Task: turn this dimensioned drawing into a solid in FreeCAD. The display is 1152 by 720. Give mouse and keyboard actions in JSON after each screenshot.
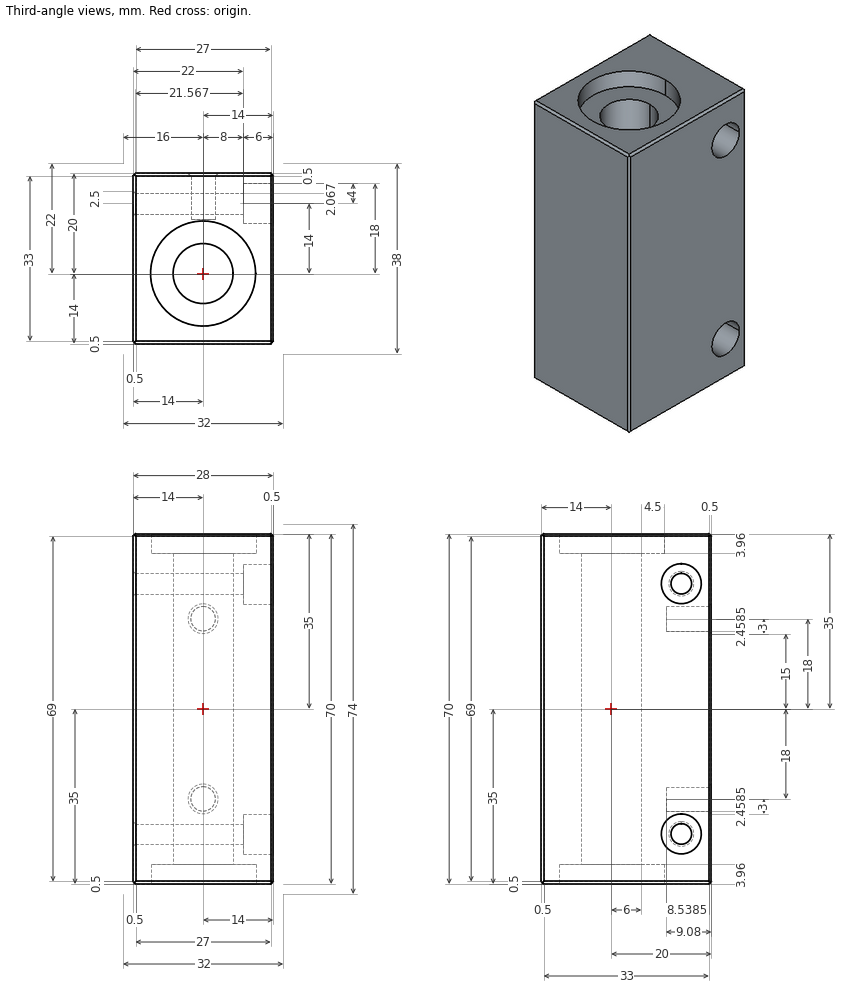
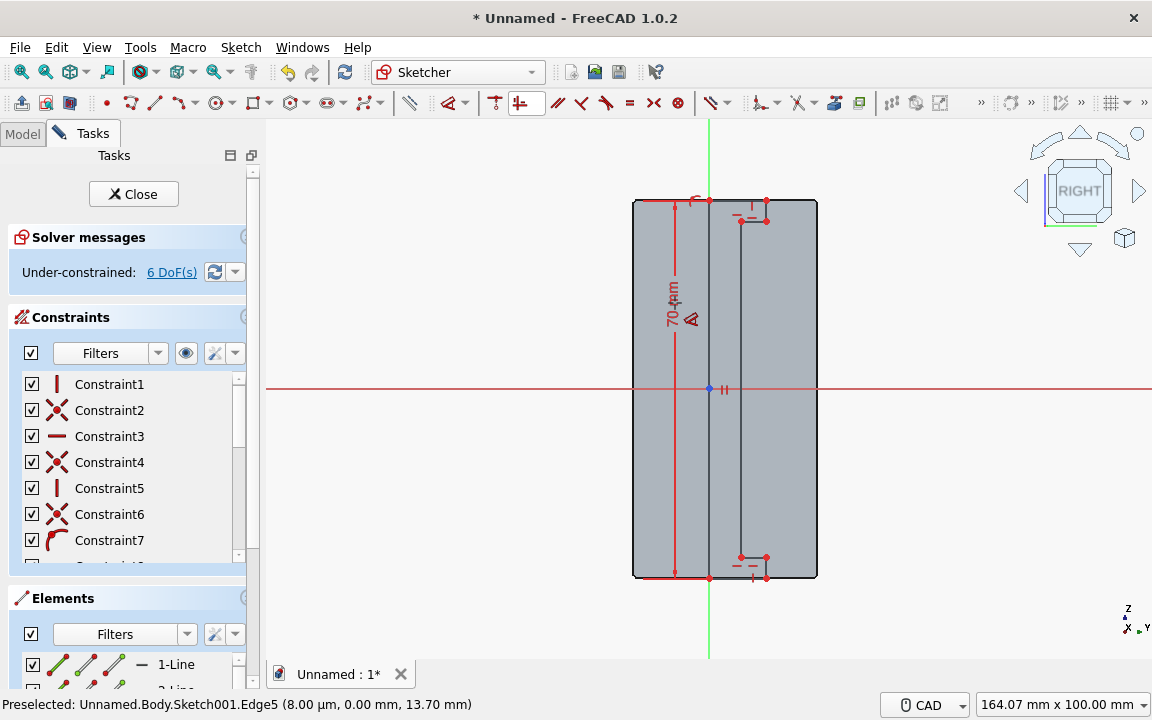
{"action": "scroll", "coordinate": [741, 558], "scroll_direction": "up", "scroll_amount": 2}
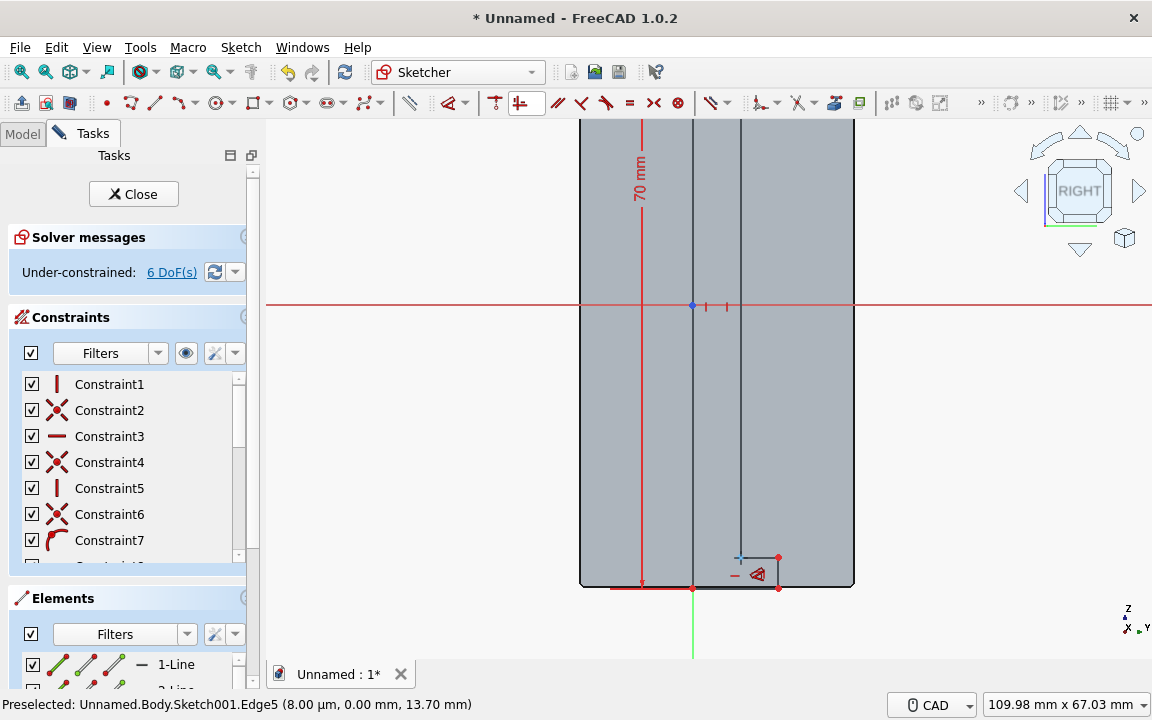
{"action": "left_click", "coordinate": [741, 558]}
{"action": "left_click", "coordinate": [717, 271]}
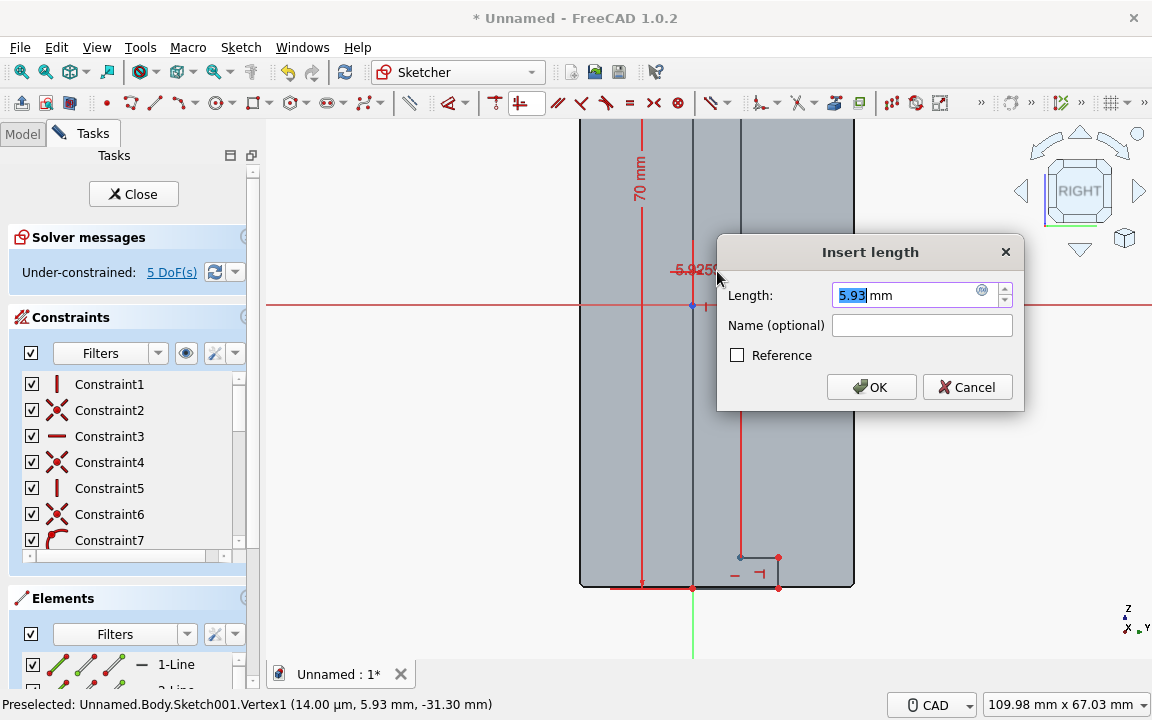
{"action": "type", "text": "6"}
{"action": "key", "text": "Return"}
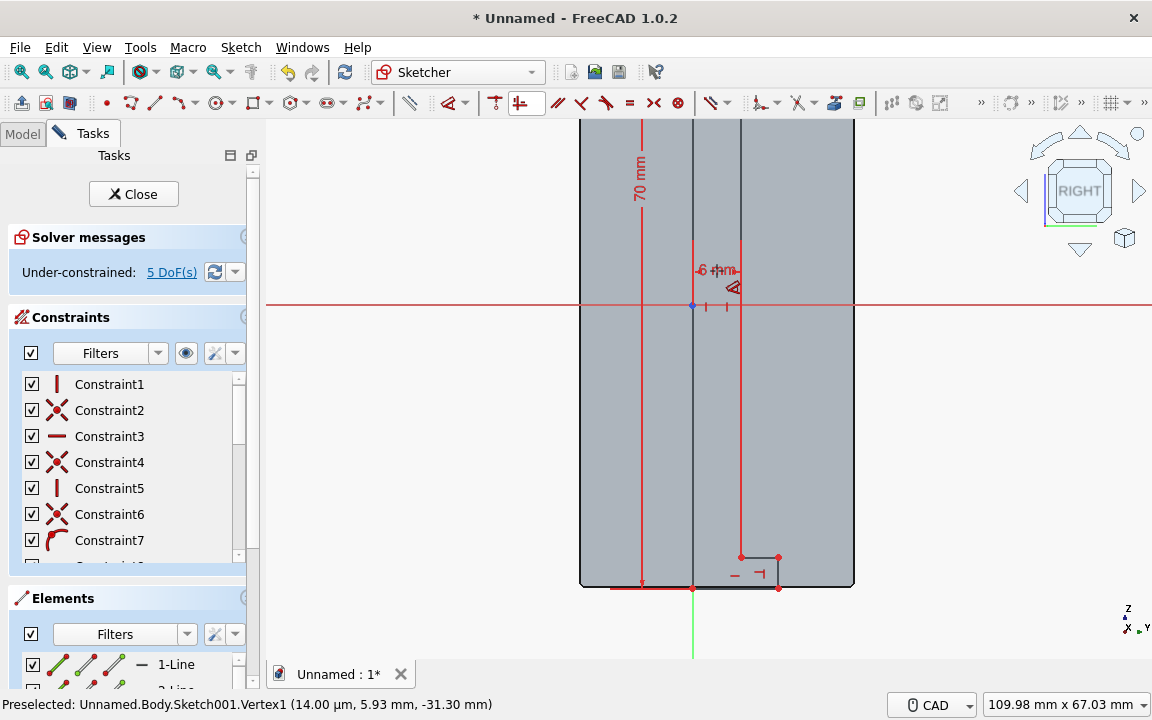
{"action": "scroll", "coordinate": [525, 491], "scroll_direction": "down", "scroll_amount": 3}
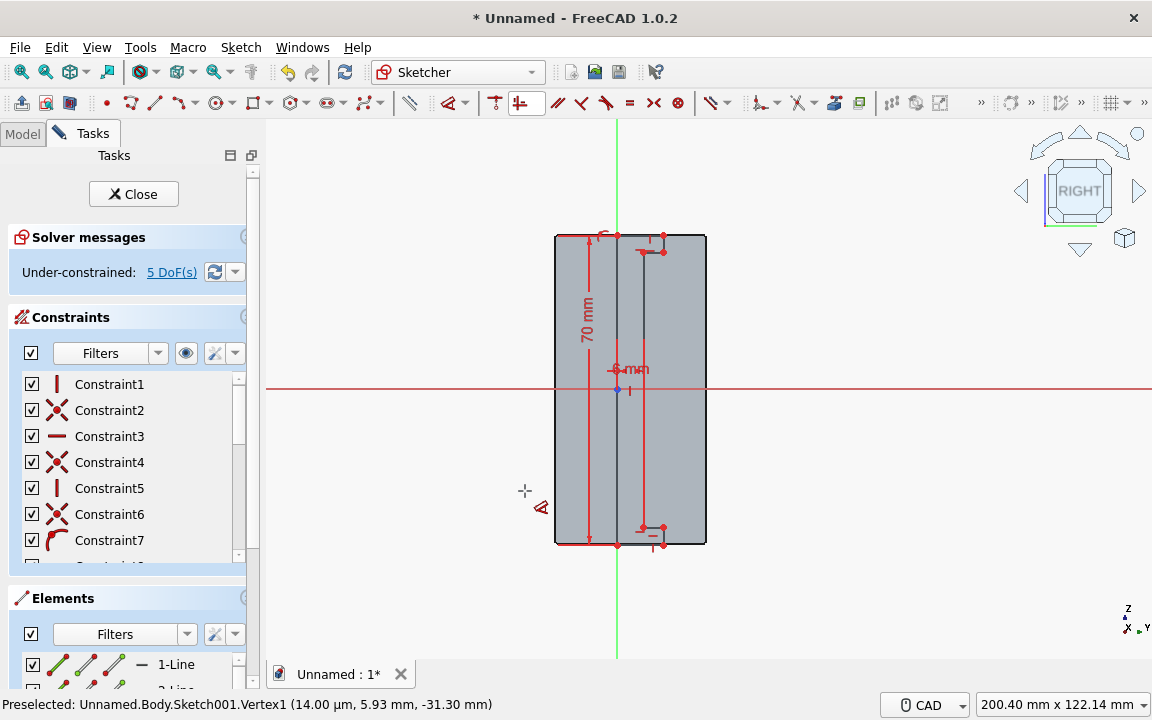
{"action": "scroll", "coordinate": [650, 253], "scroll_direction": "up", "scroll_amount": 5}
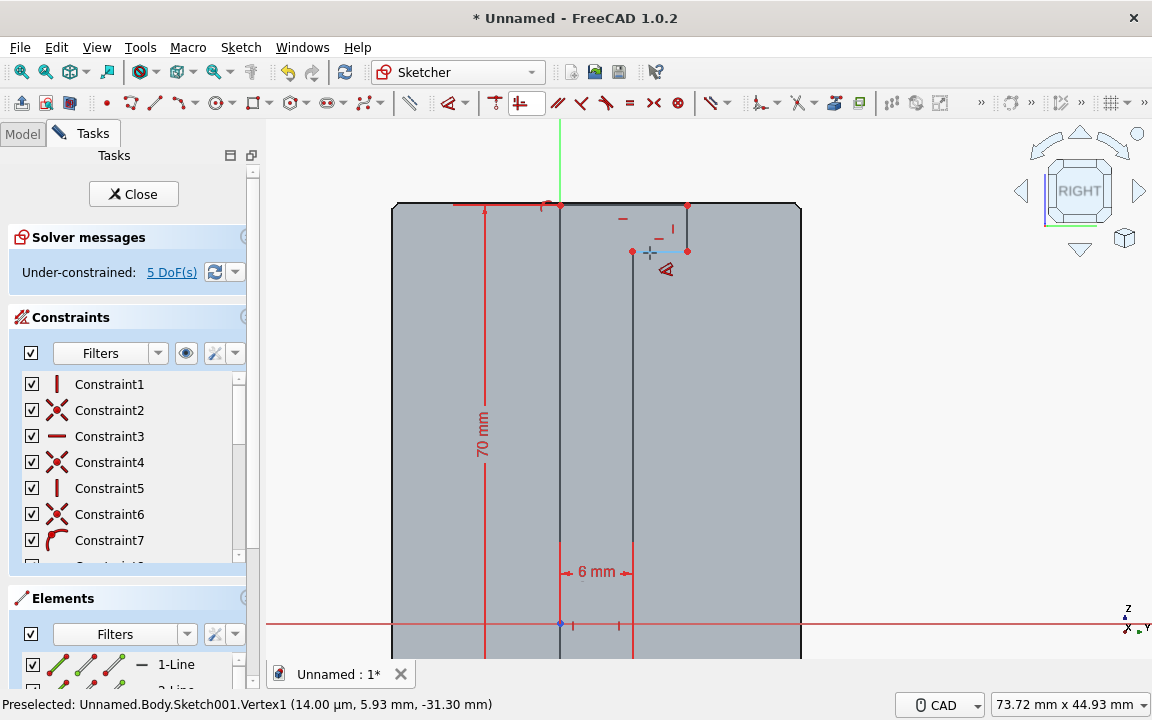
{"action": "left_click", "coordinate": [649, 252]}
{"action": "left_click", "coordinate": [660, 286]}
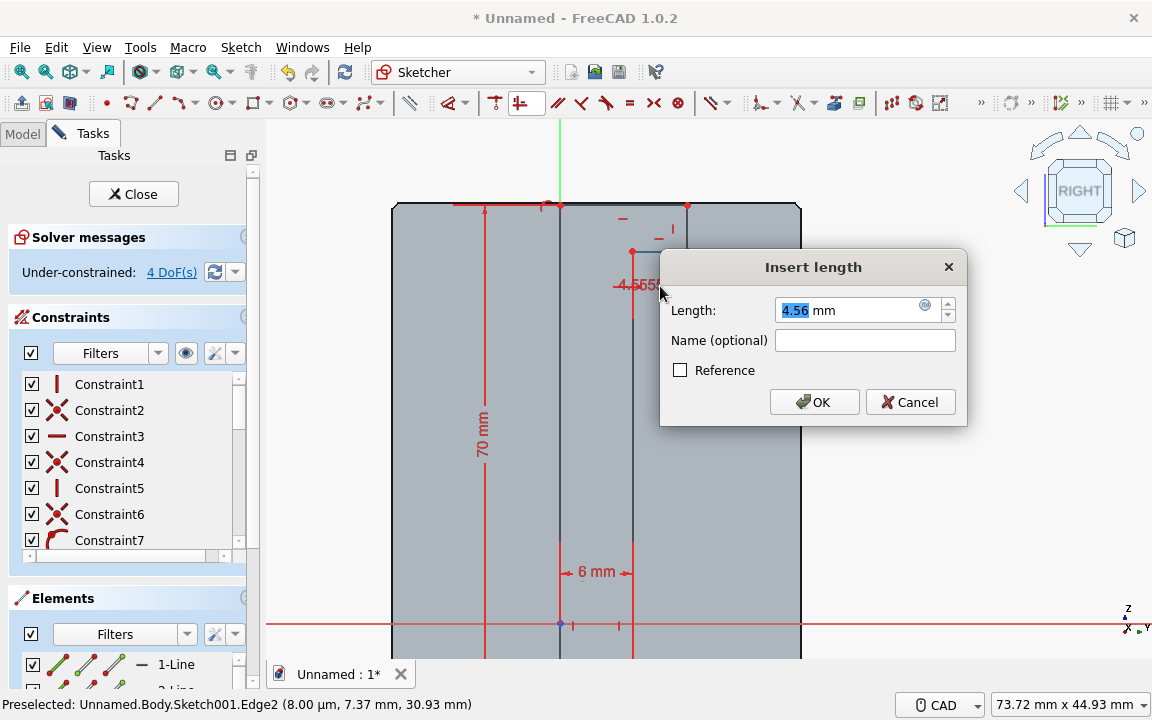
{"action": "type", "text": "4.5"}
{"action": "key", "text": "Return"}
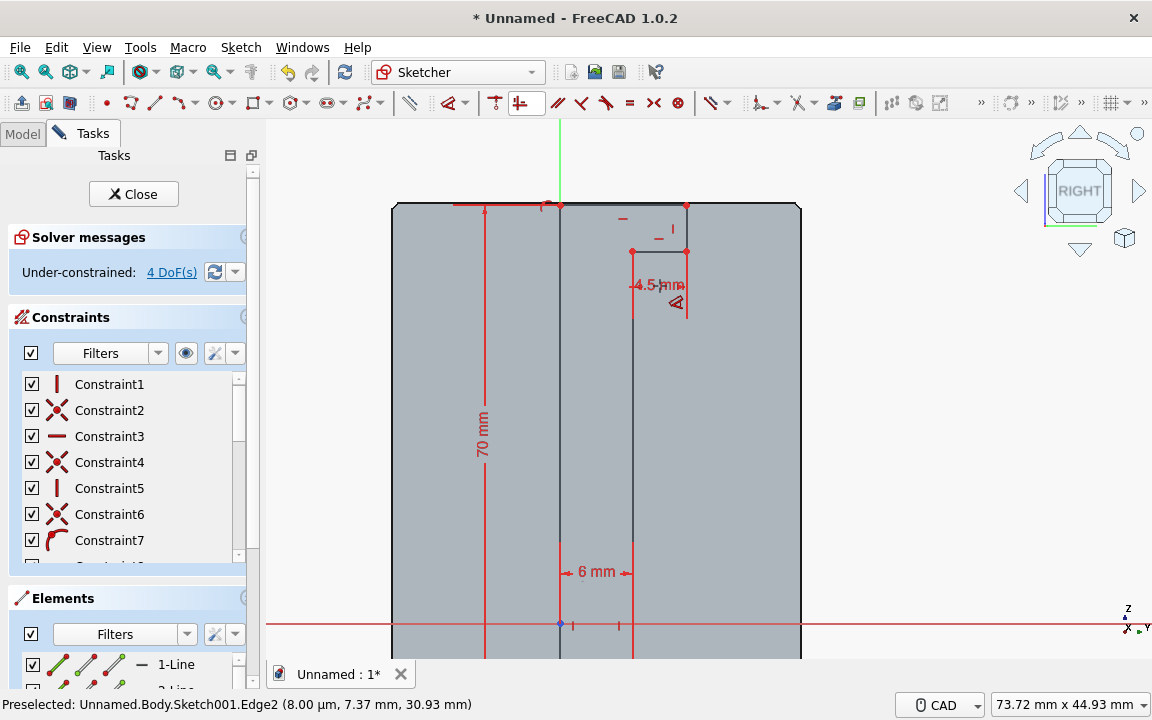
{"action": "scroll", "coordinate": [650, 252], "scroll_direction": "down", "scroll_amount": 5}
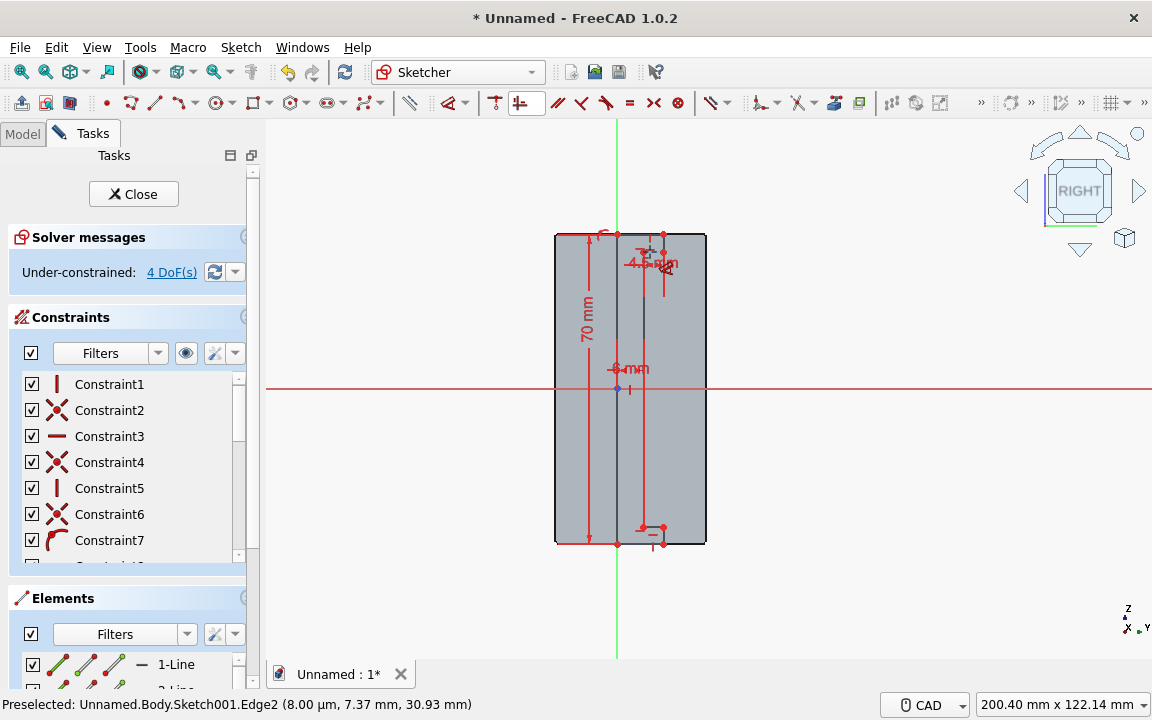
{"action": "scroll", "coordinate": [658, 527], "scroll_direction": "up", "scroll_amount": 5}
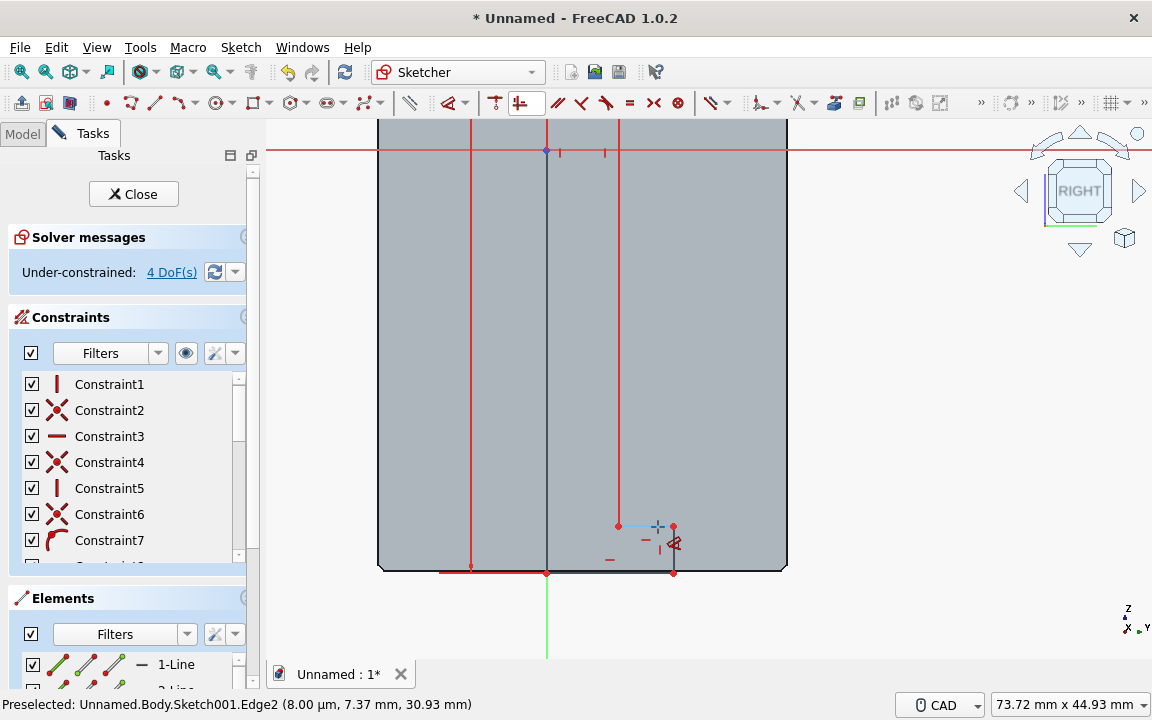
{"action": "left_click", "coordinate": [657, 526]}
{"action": "left_click", "coordinate": [646, 492]}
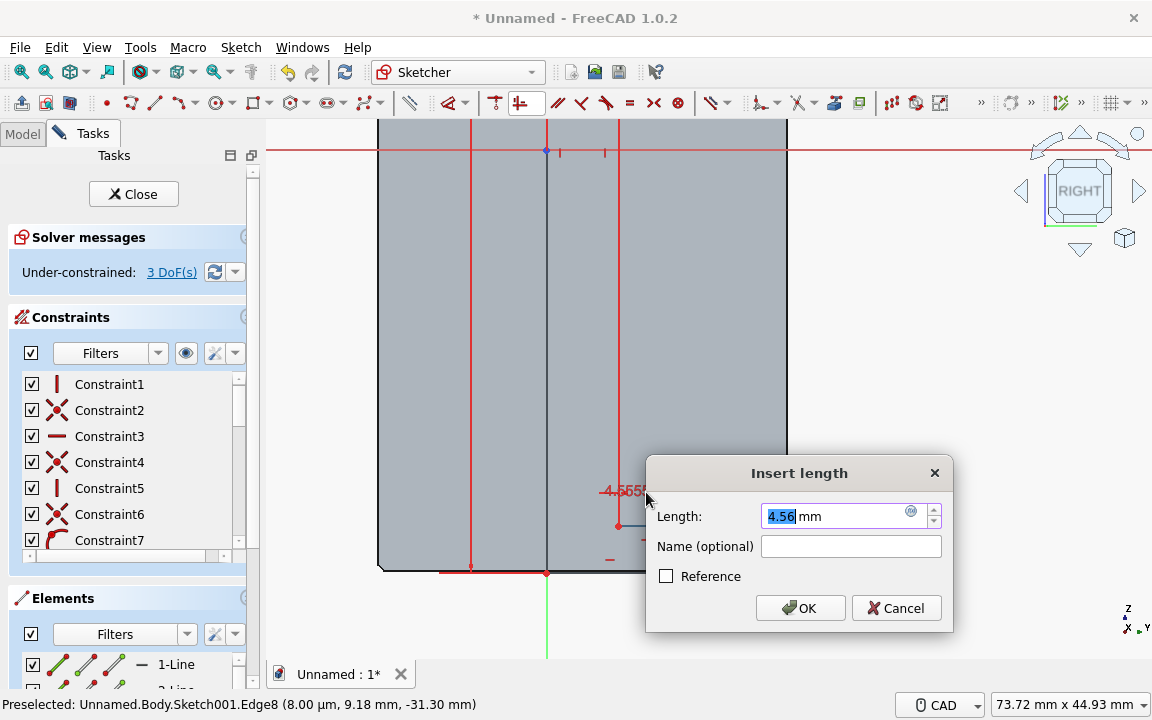
{"action": "type", "text": "4.5"}
{"action": "key", "text": "Return"}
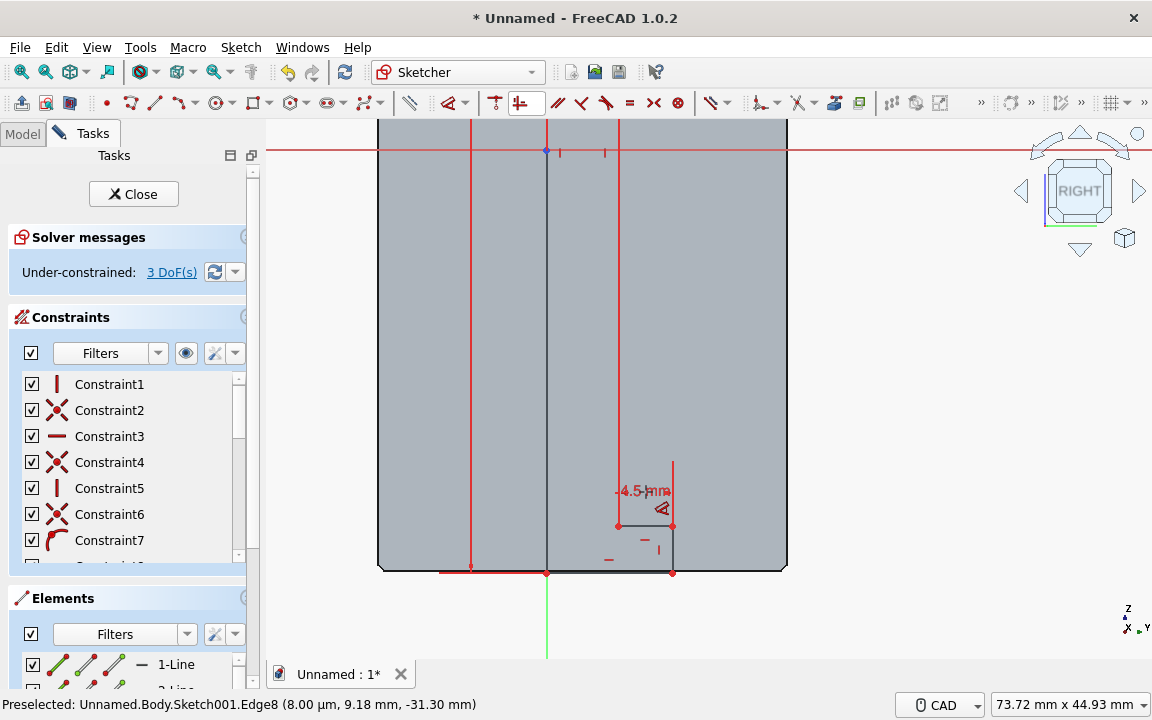
{"action": "scroll", "coordinate": [658, 528], "scroll_direction": "down", "scroll_amount": 5}